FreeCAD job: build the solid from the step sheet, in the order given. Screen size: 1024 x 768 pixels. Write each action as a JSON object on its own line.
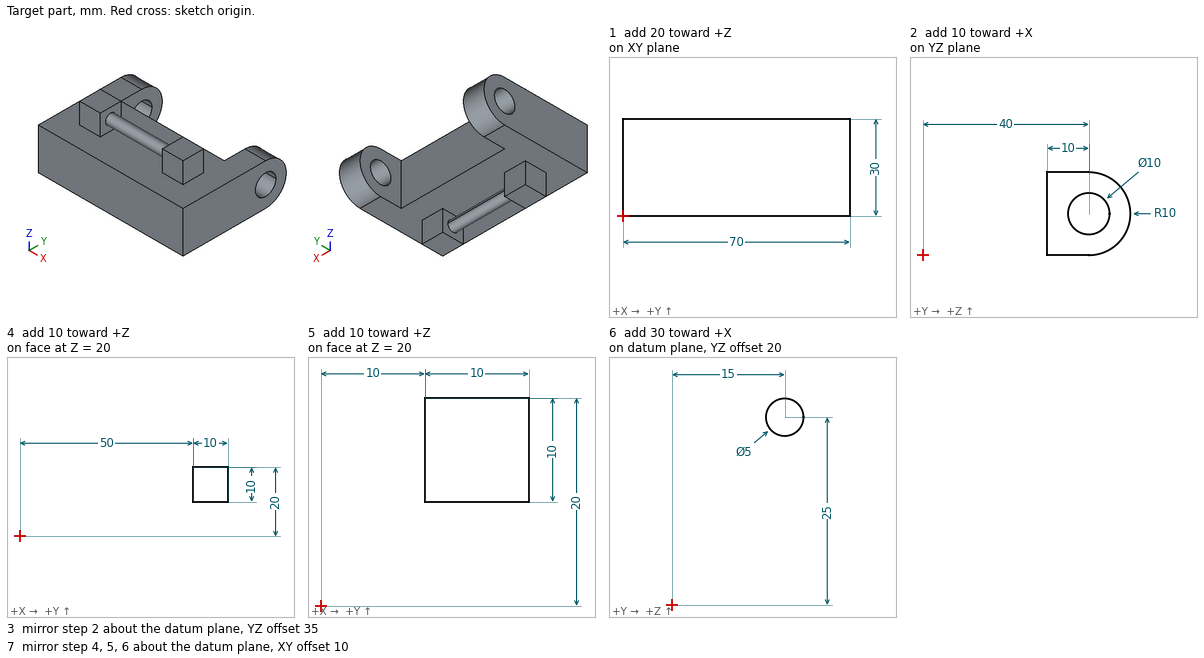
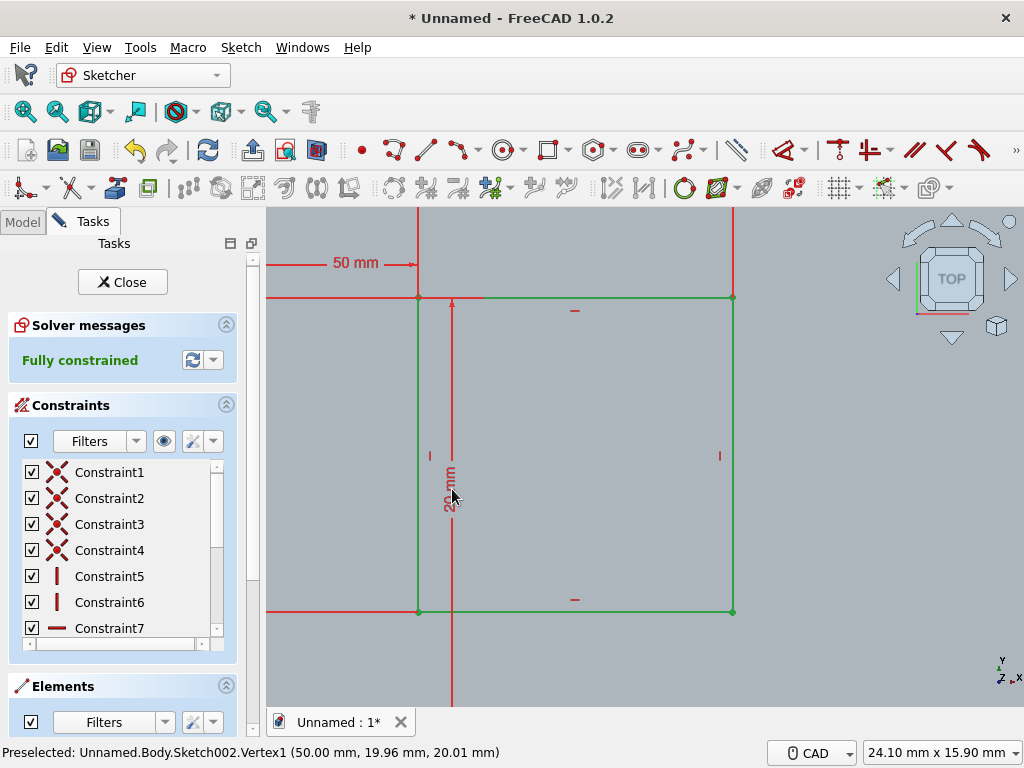
{"action": "left_click", "coordinate": [123, 282]}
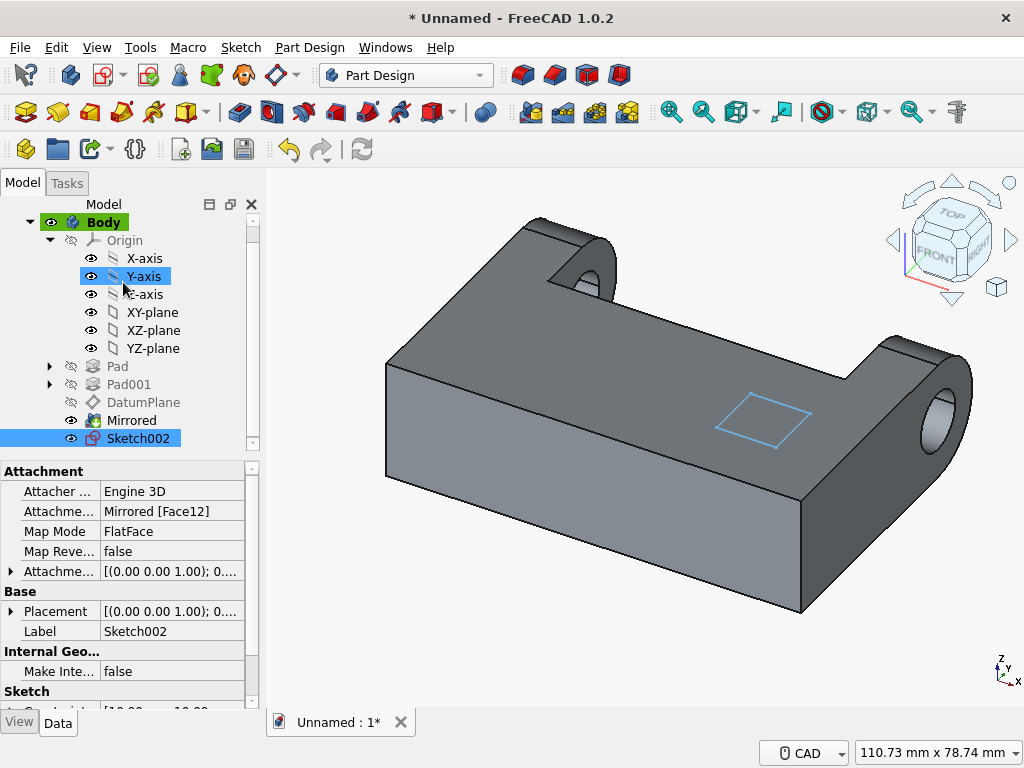
{"action": "left_click", "coordinate": [26, 112]}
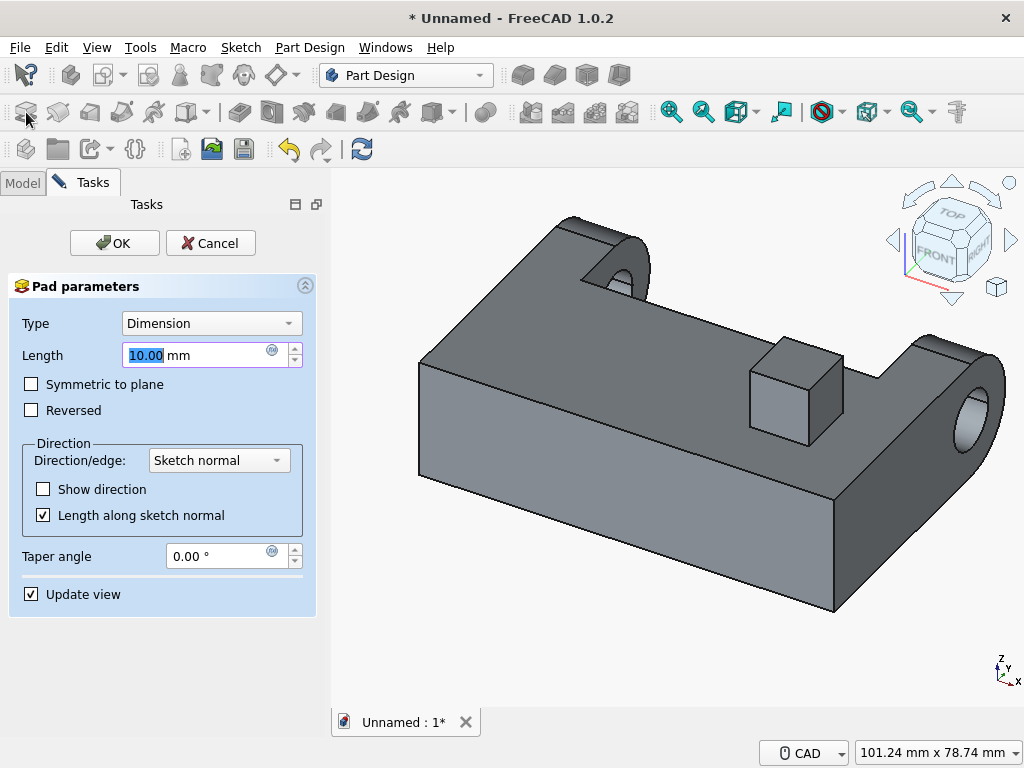
{"action": "type", "text": "10"}
{"action": "key", "text": "Tab"}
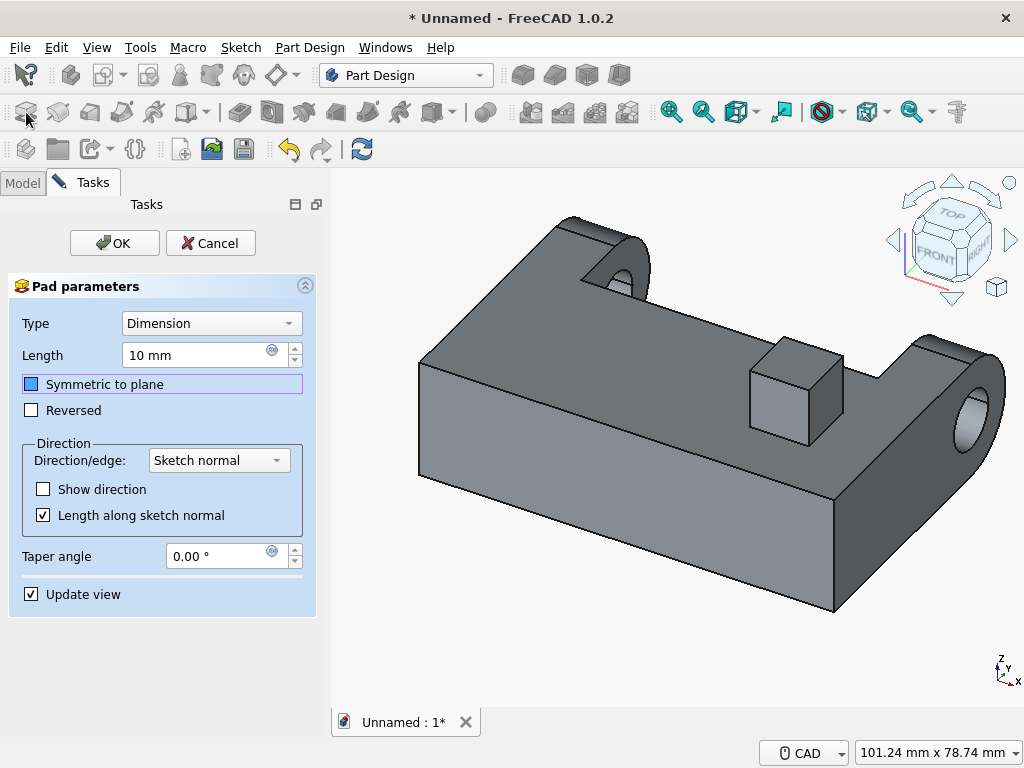
{"action": "left_click", "coordinate": [115, 243]}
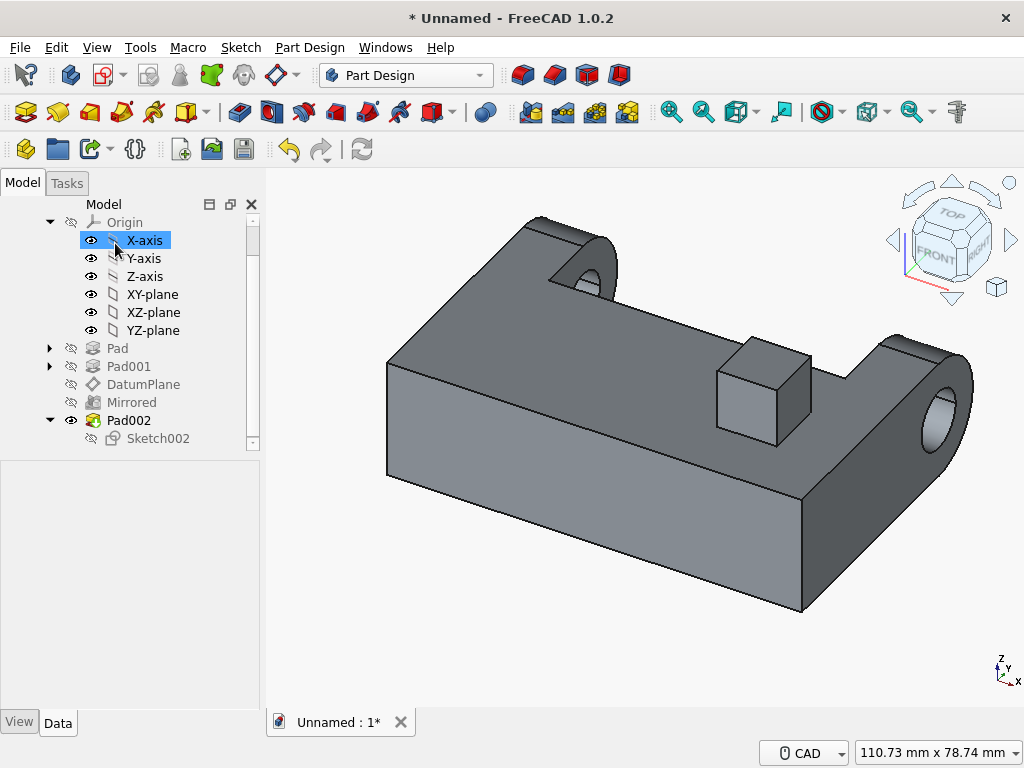
{"action": "key", "text": "v f"}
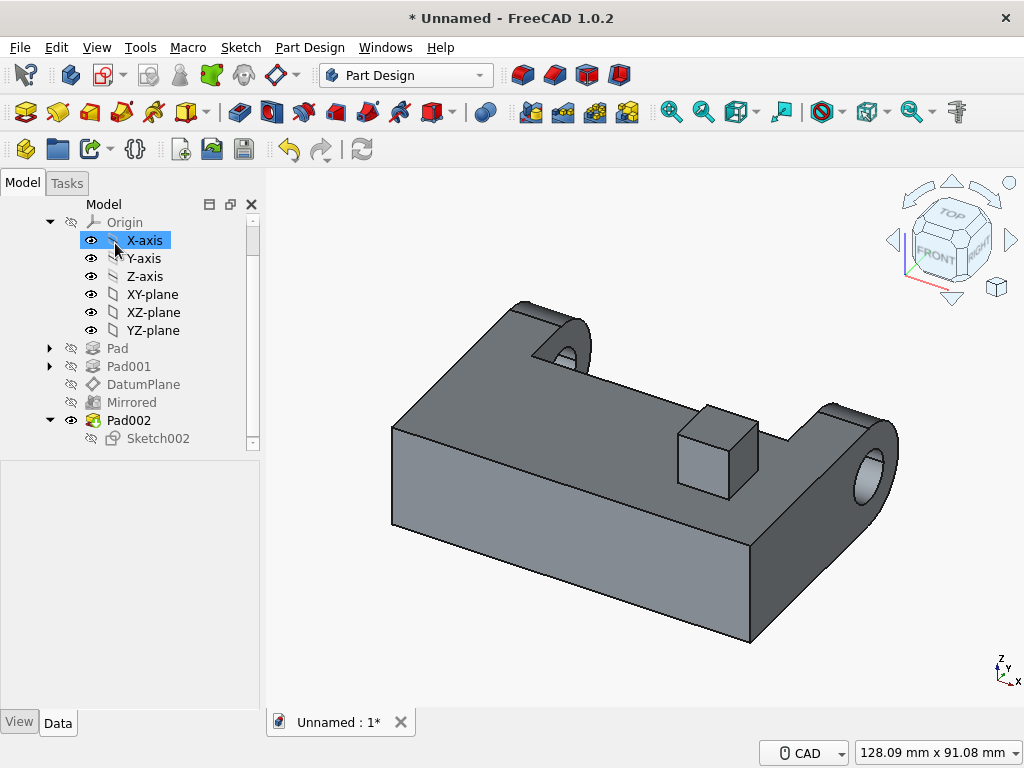
{"action": "left_click", "coordinate": [613, 444]}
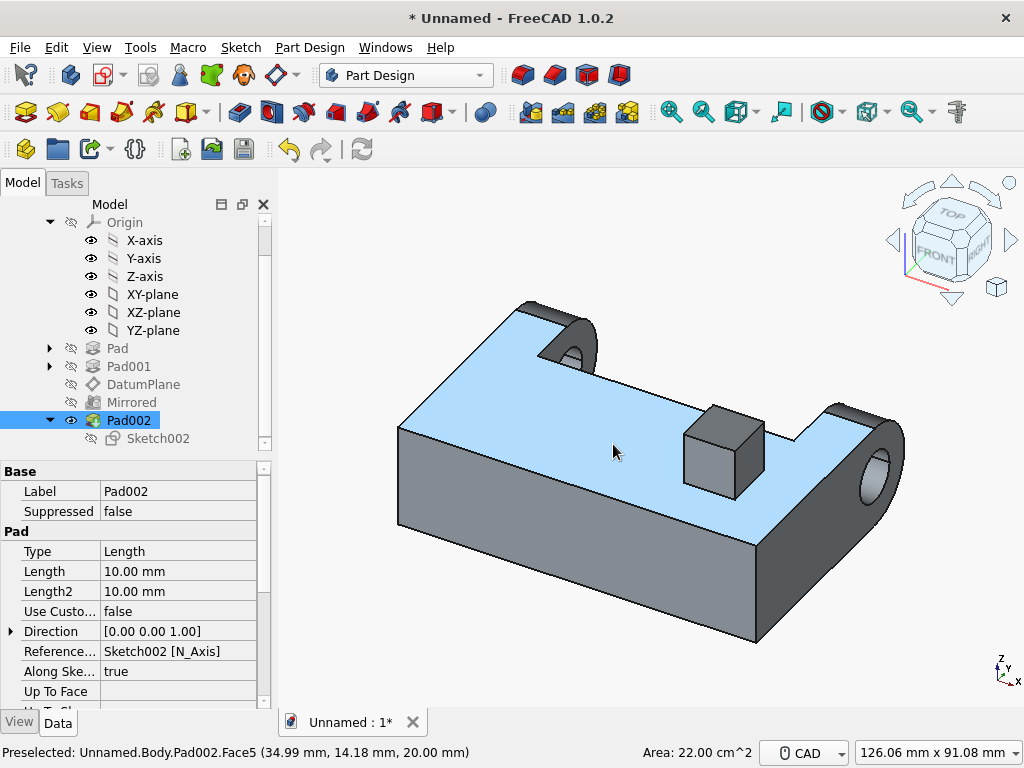
{"action": "left_click", "coordinate": [104, 76]}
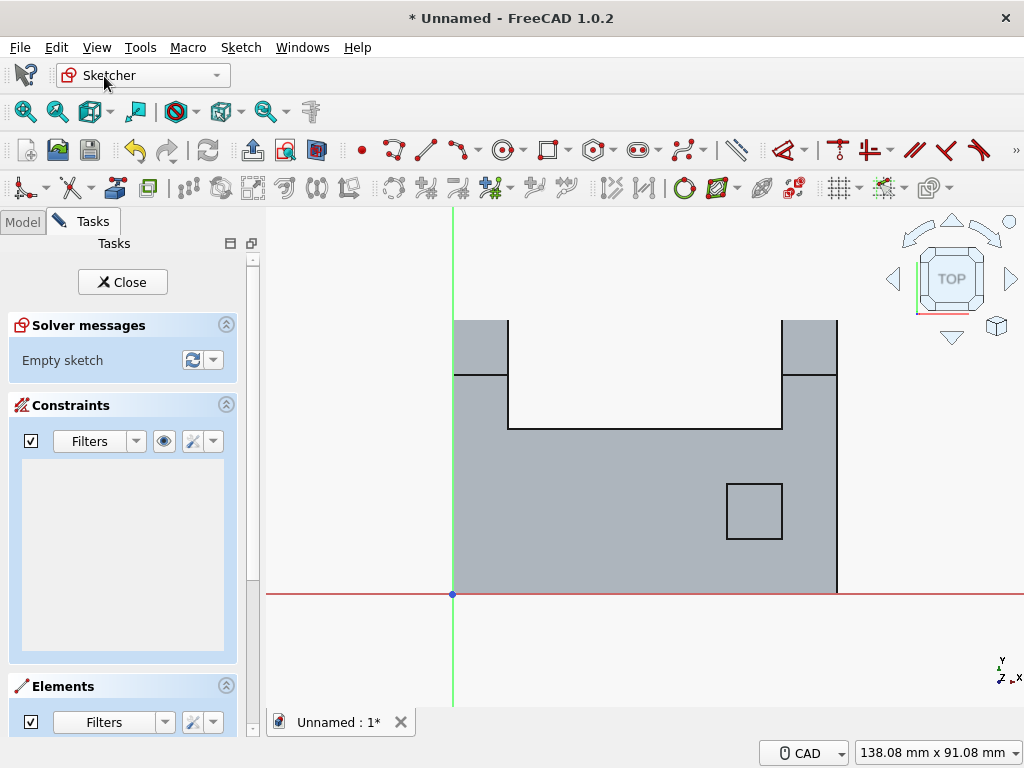
{"action": "scroll", "coordinate": [468, 587], "scroll_direction": "up", "scroll_amount": 5}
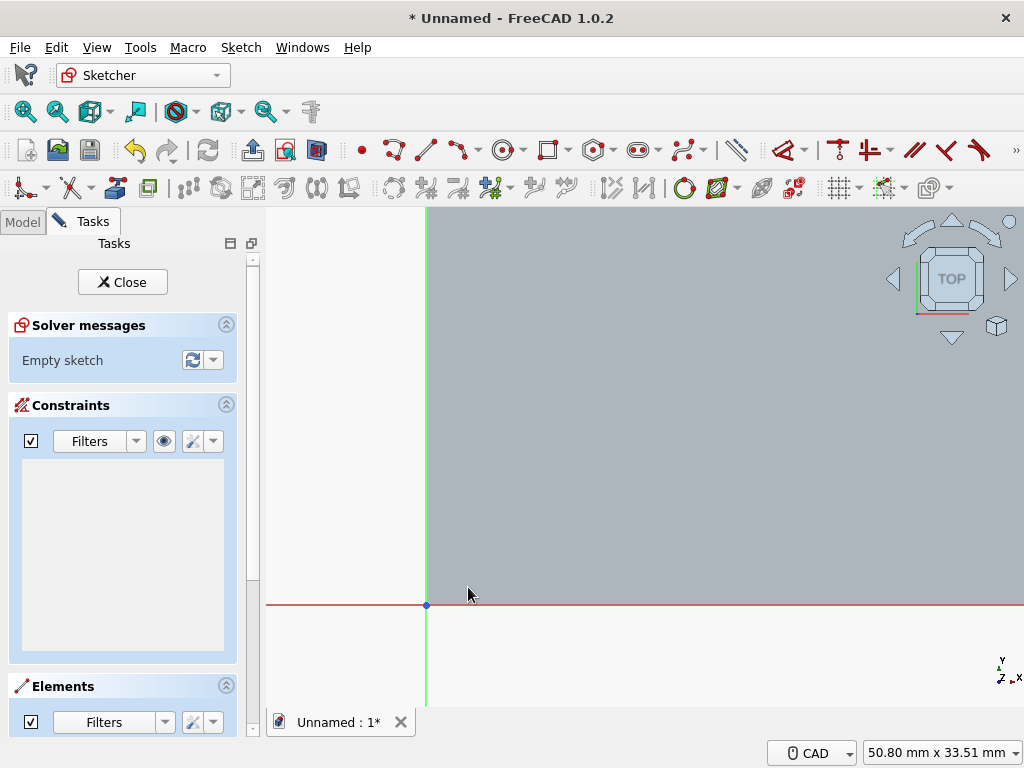
{"action": "key", "text": "g r"}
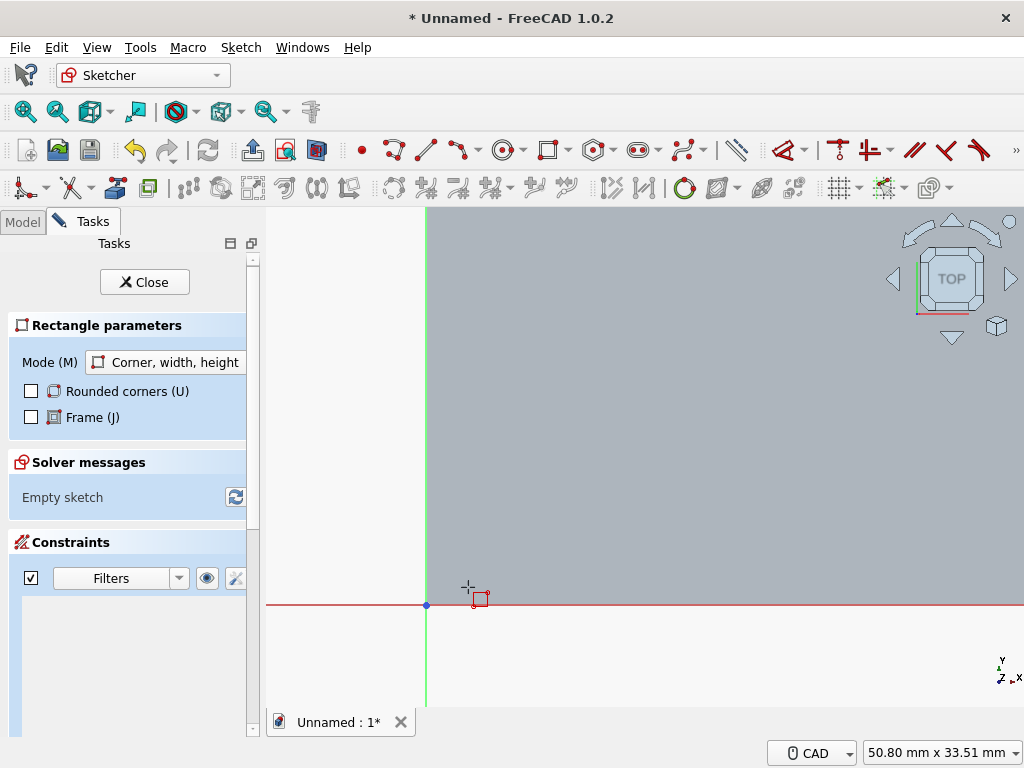
{"action": "left_click", "coordinate": [576, 307]}
{"action": "mouse_move", "coordinate": [725, 456]}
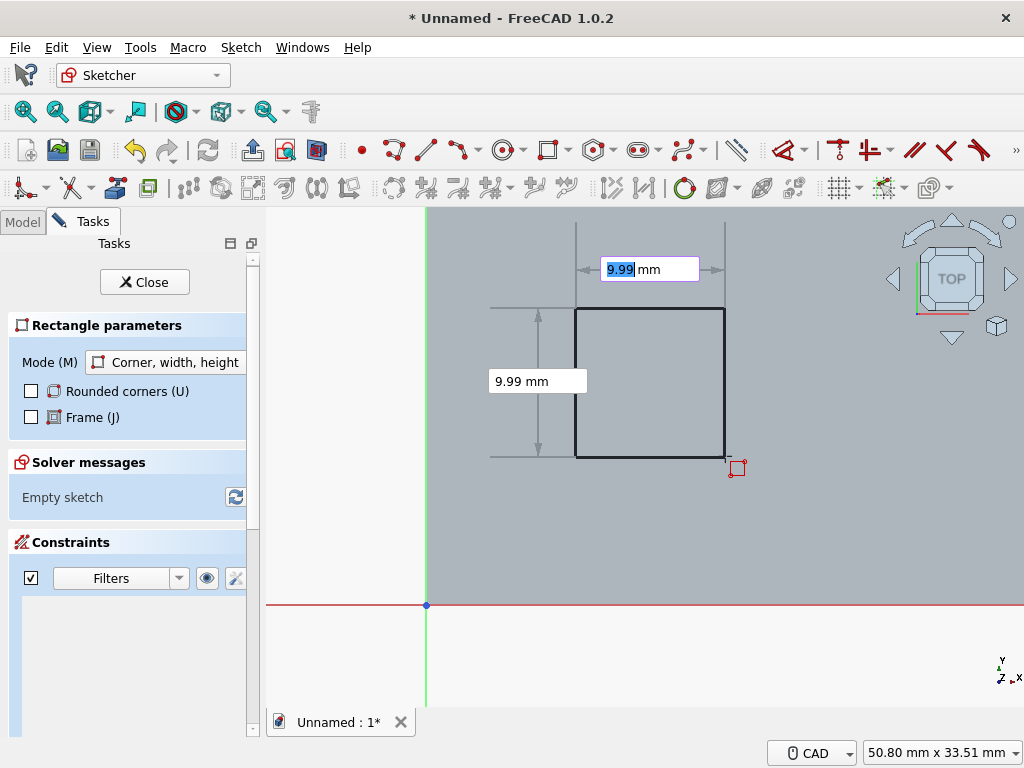
{"action": "type", "text": "10"}
{"action": "key", "text": "Tab"}
{"action": "type", "text": "10"}
{"action": "key", "text": "Return"}
{"action": "key", "text": "Escape"}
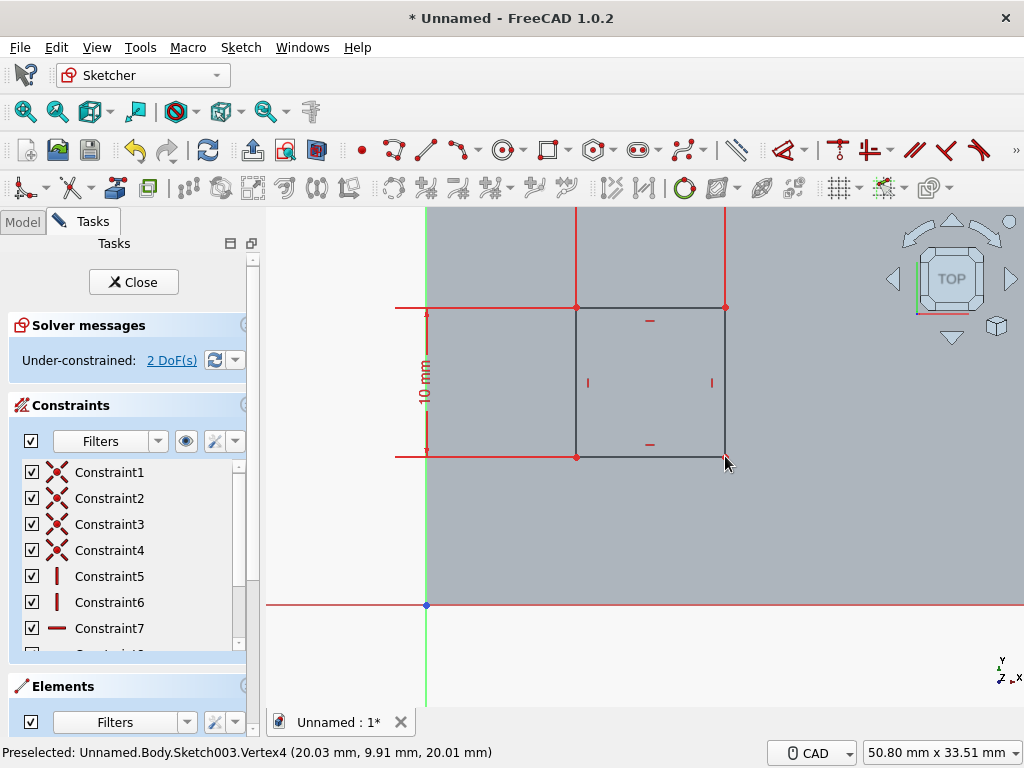
{"action": "key", "text": "d"}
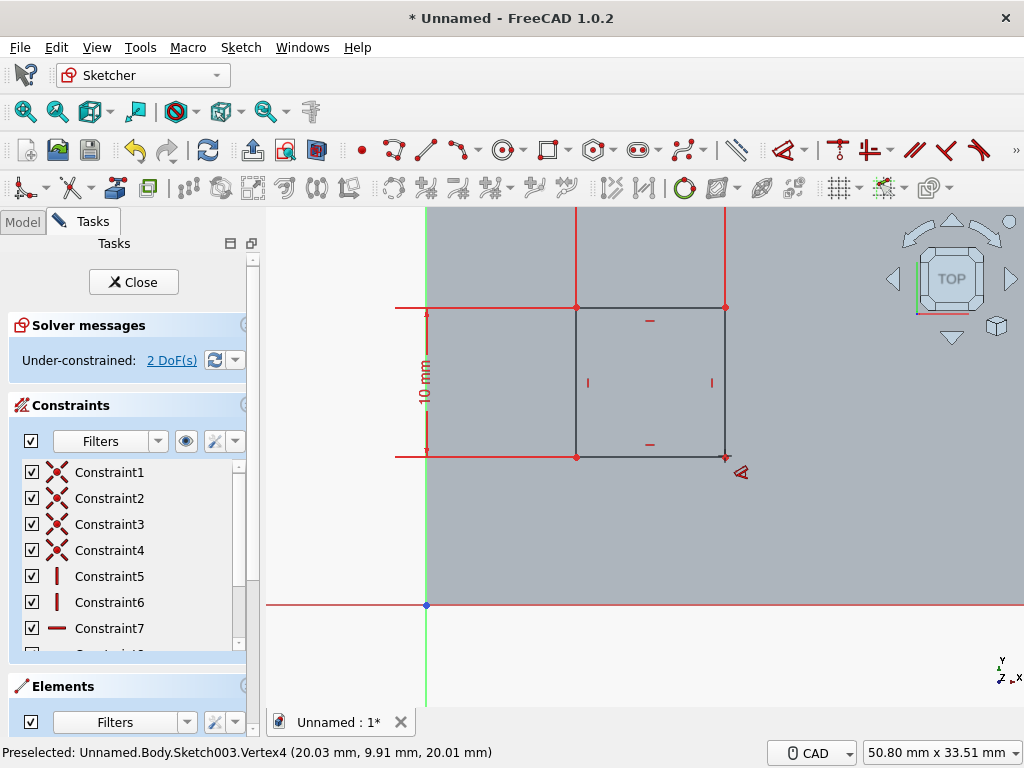
{"action": "left_click", "coordinate": [576, 308]}
{"action": "left_click", "coordinate": [501, 639]}